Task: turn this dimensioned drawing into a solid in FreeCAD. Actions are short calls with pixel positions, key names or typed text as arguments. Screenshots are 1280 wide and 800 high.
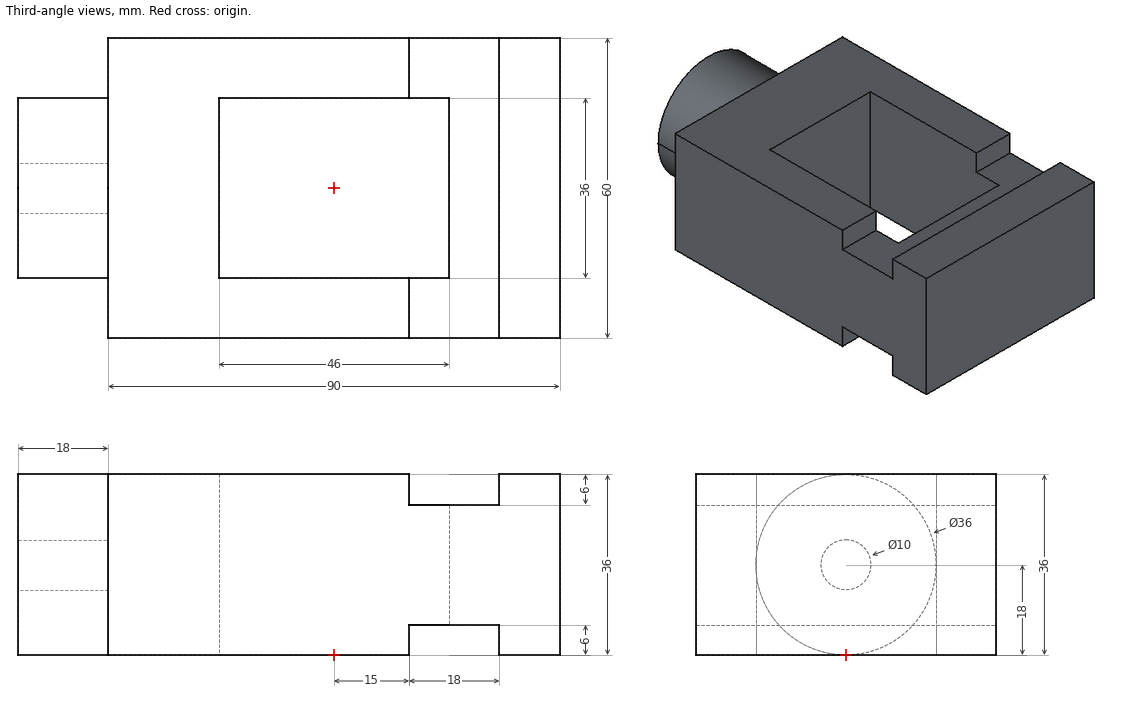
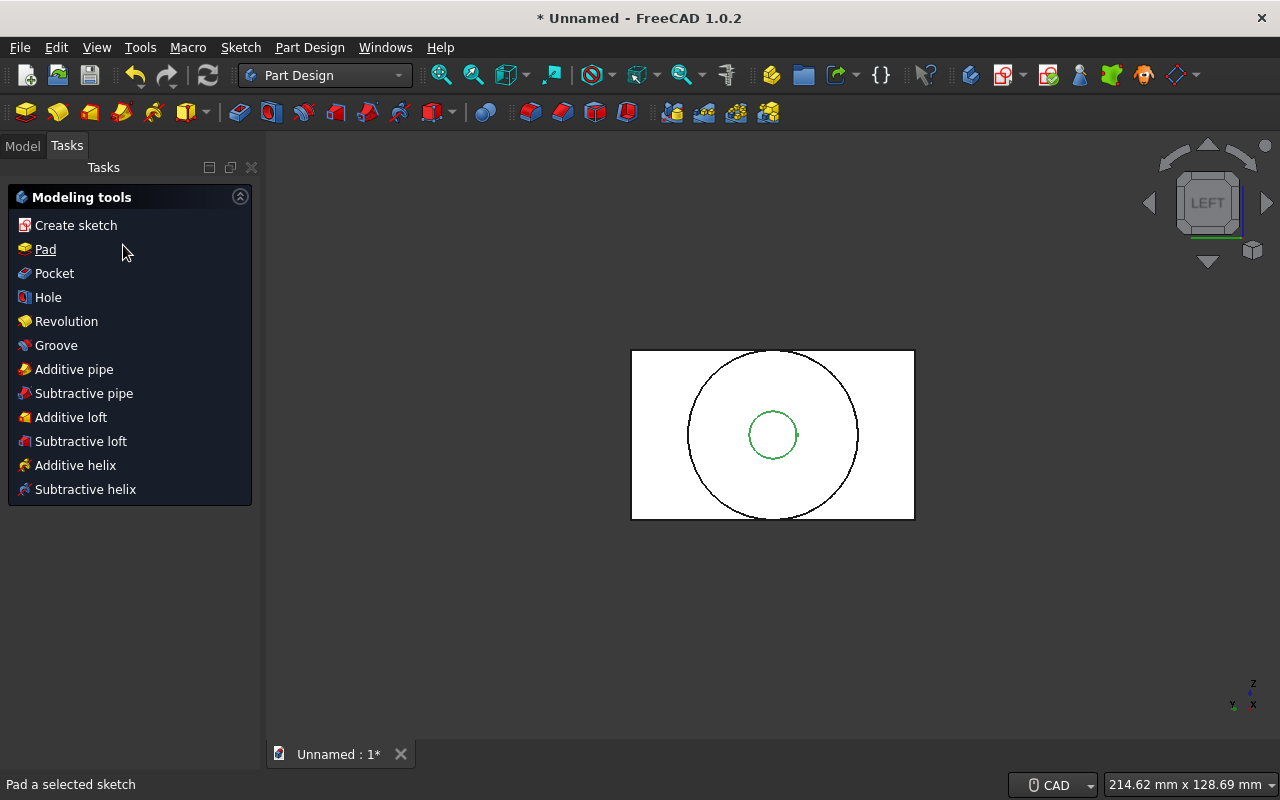
click(240, 112)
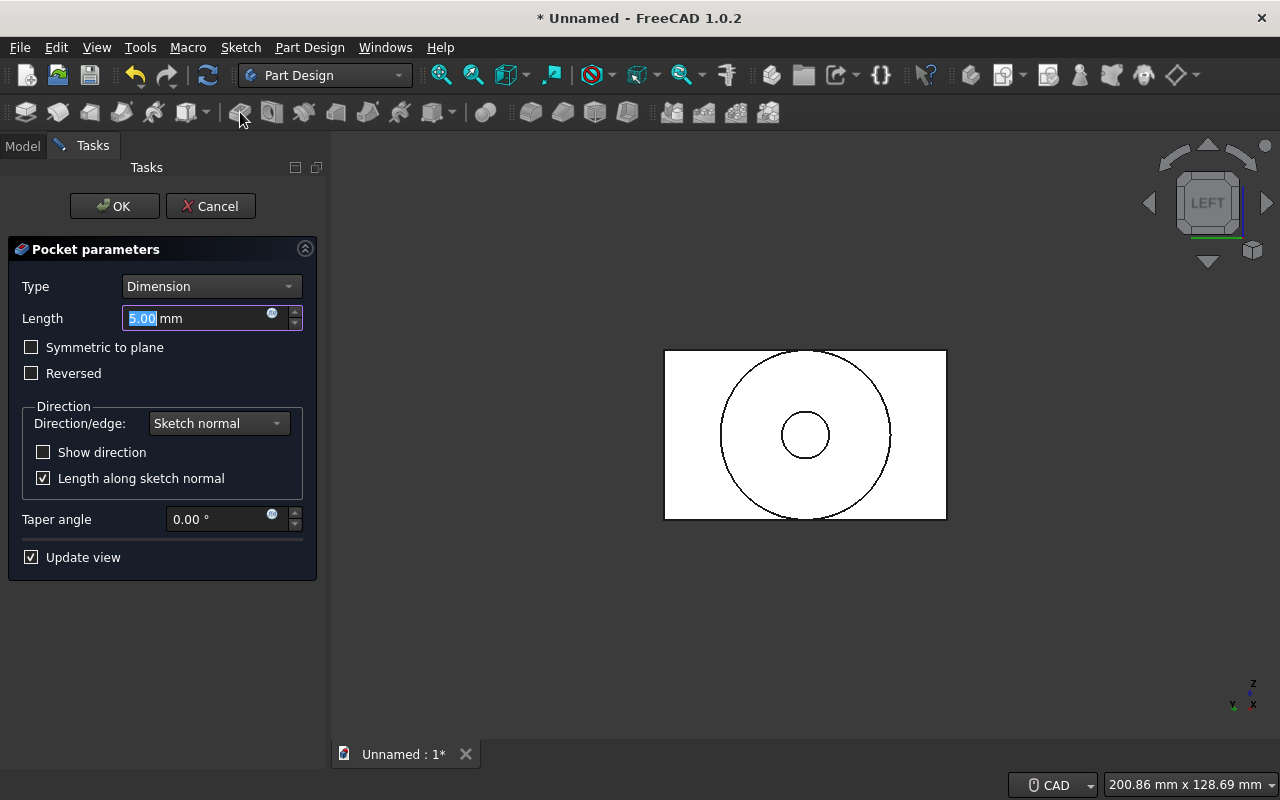
text(18)
key(Tab)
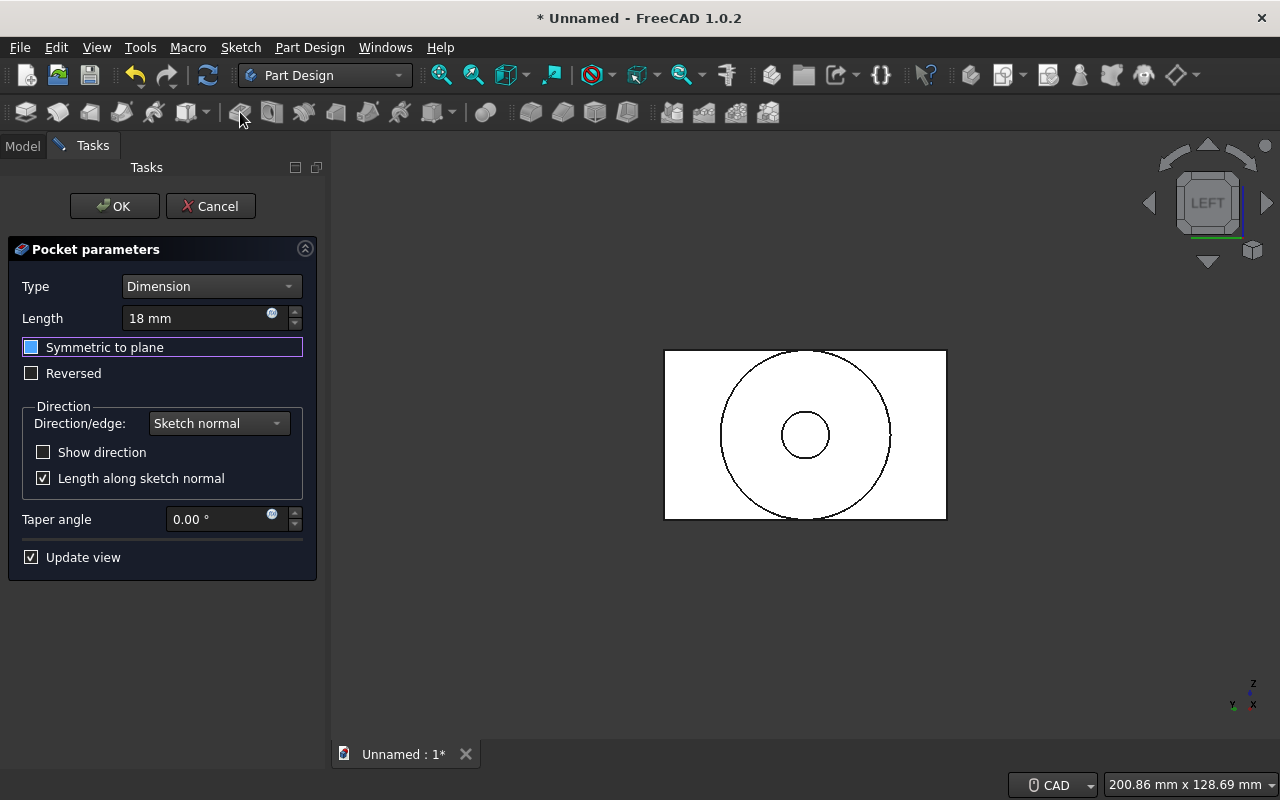
click(115, 206)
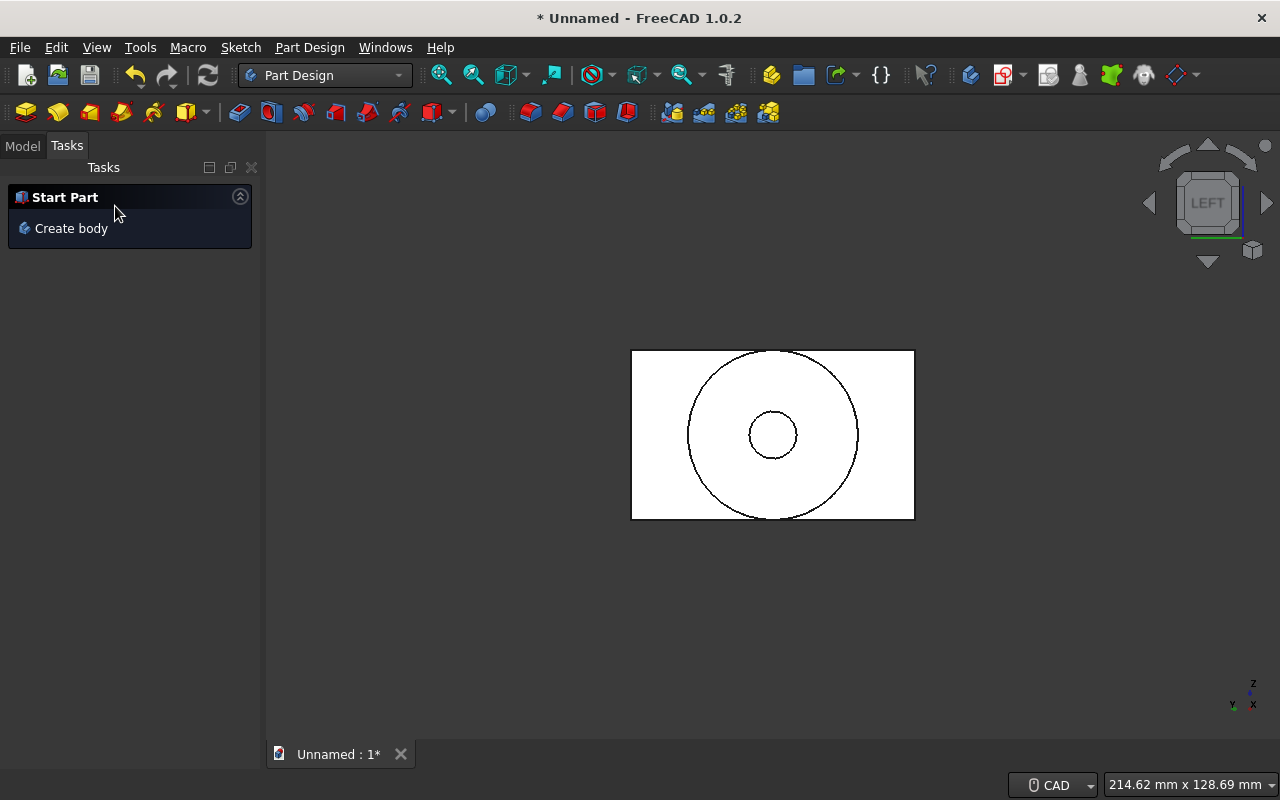
click(442, 76)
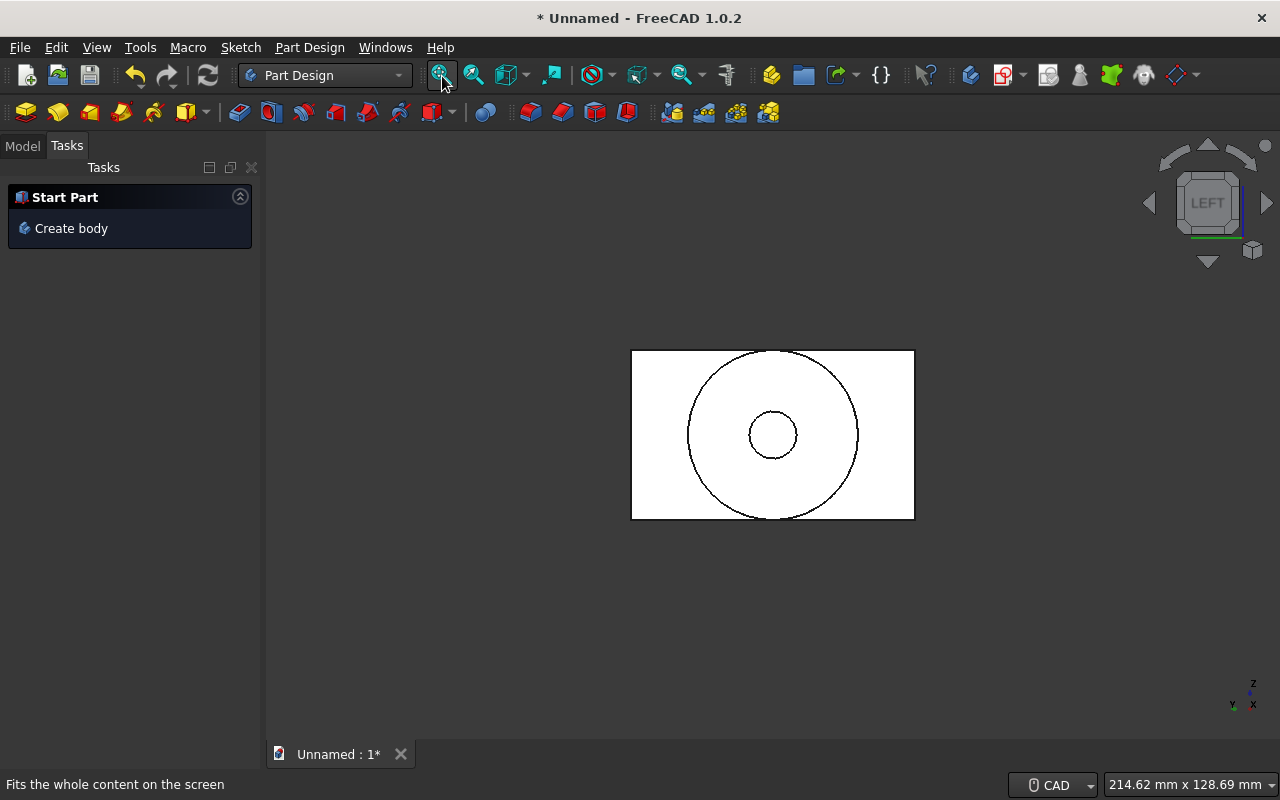
key(0)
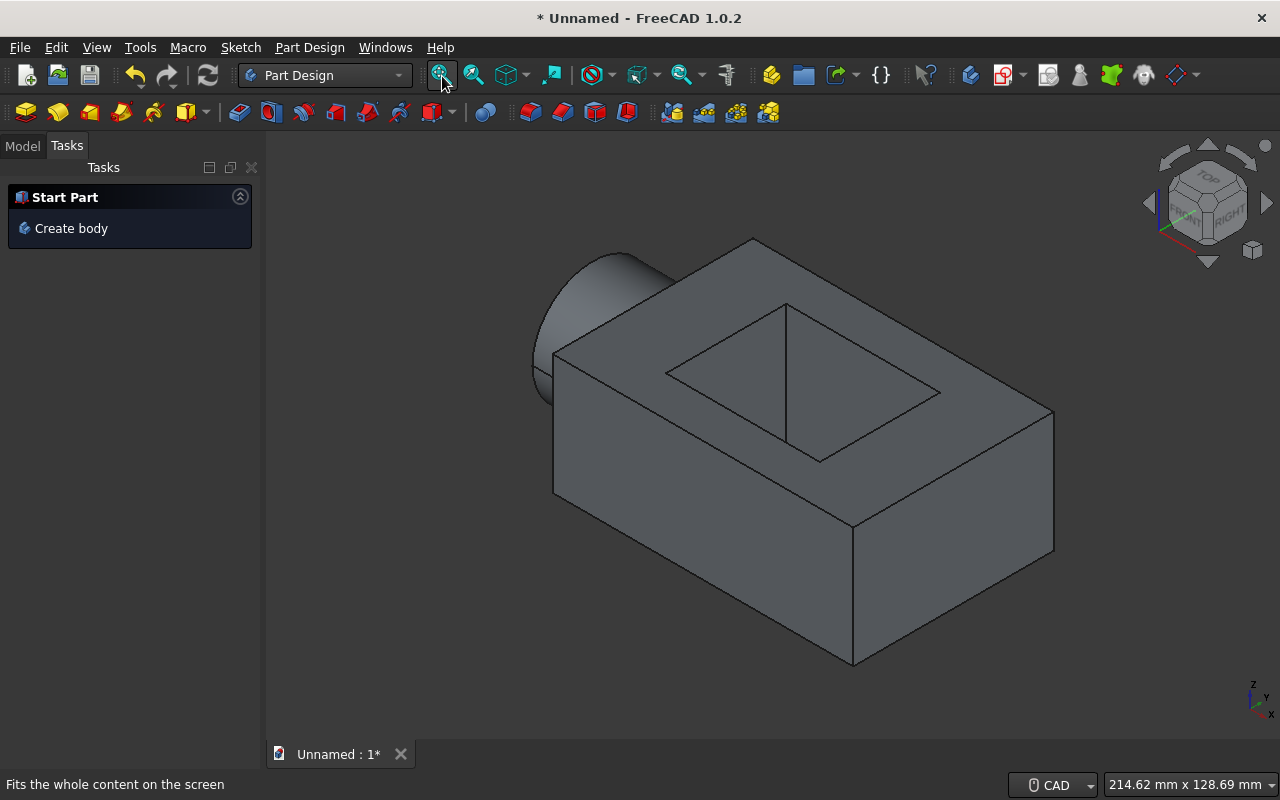
click(789, 559)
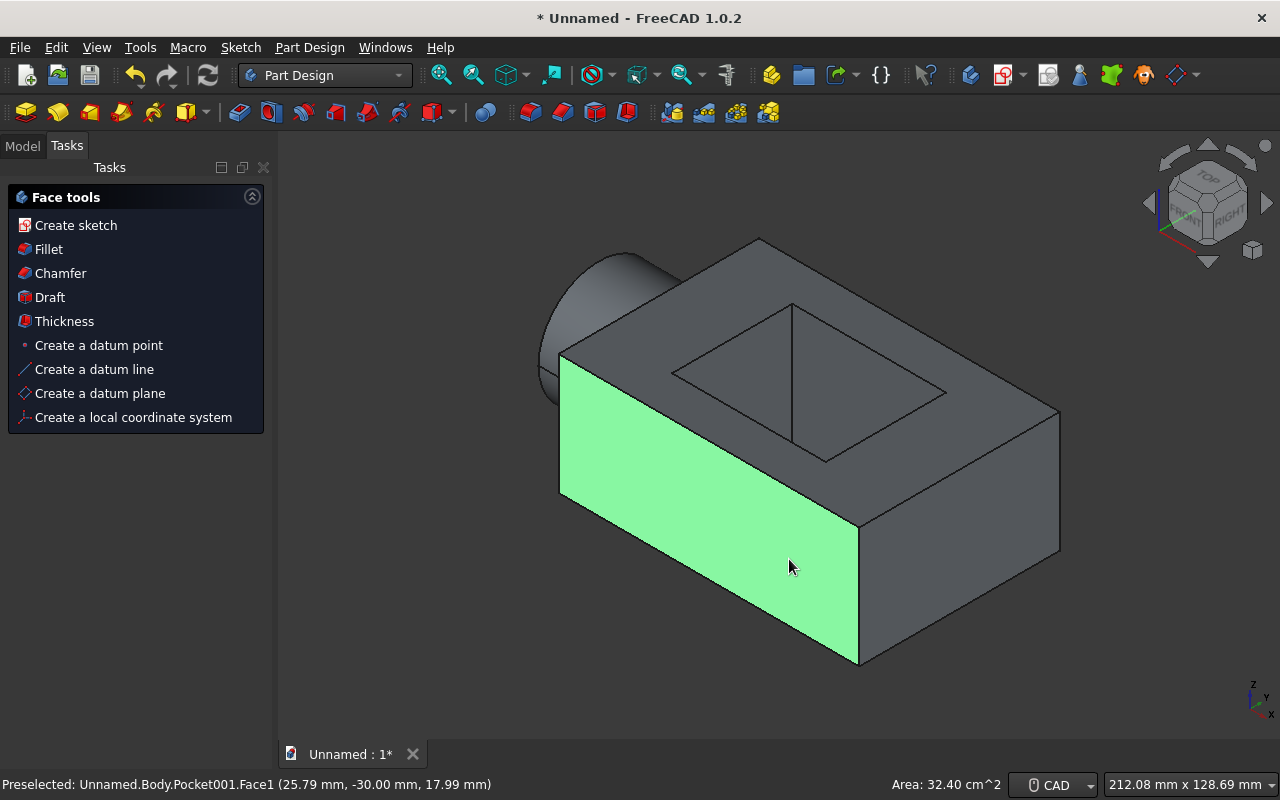
click(1004, 76)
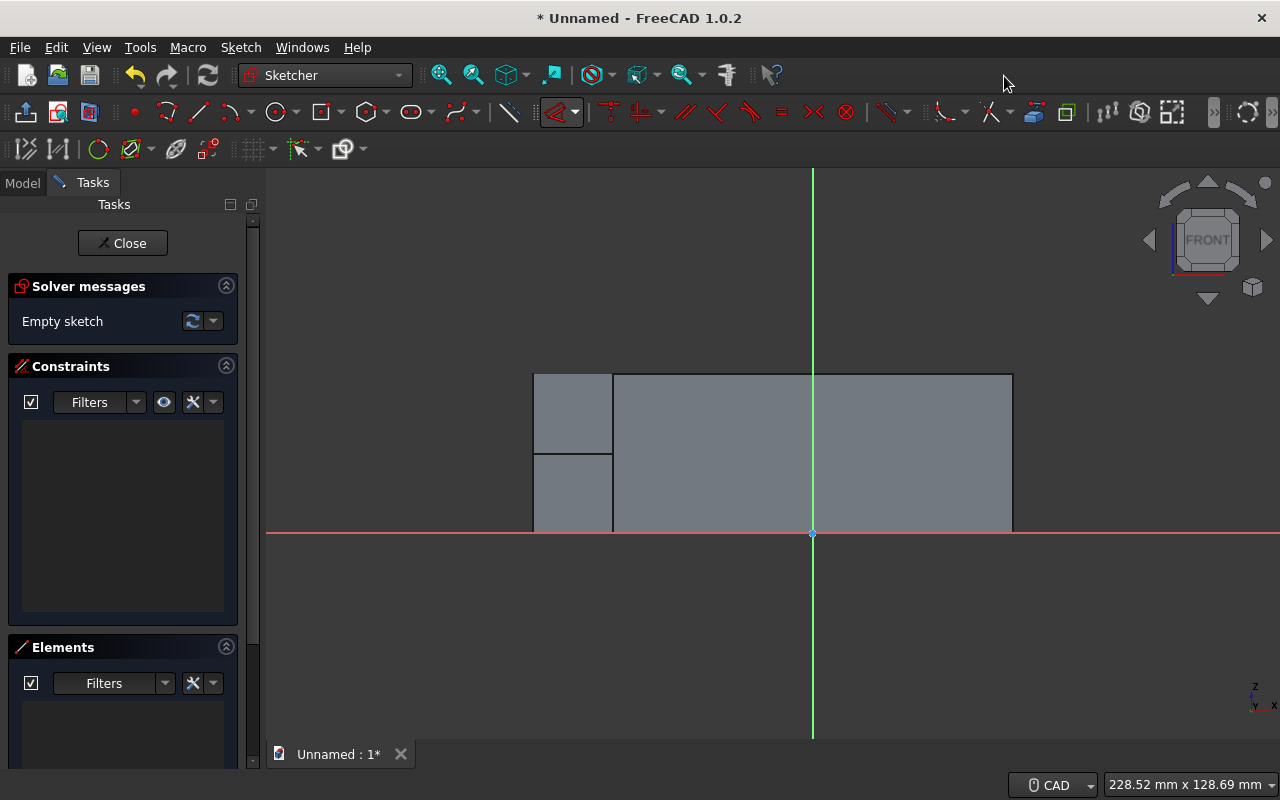
scroll(946, 542, up, 7)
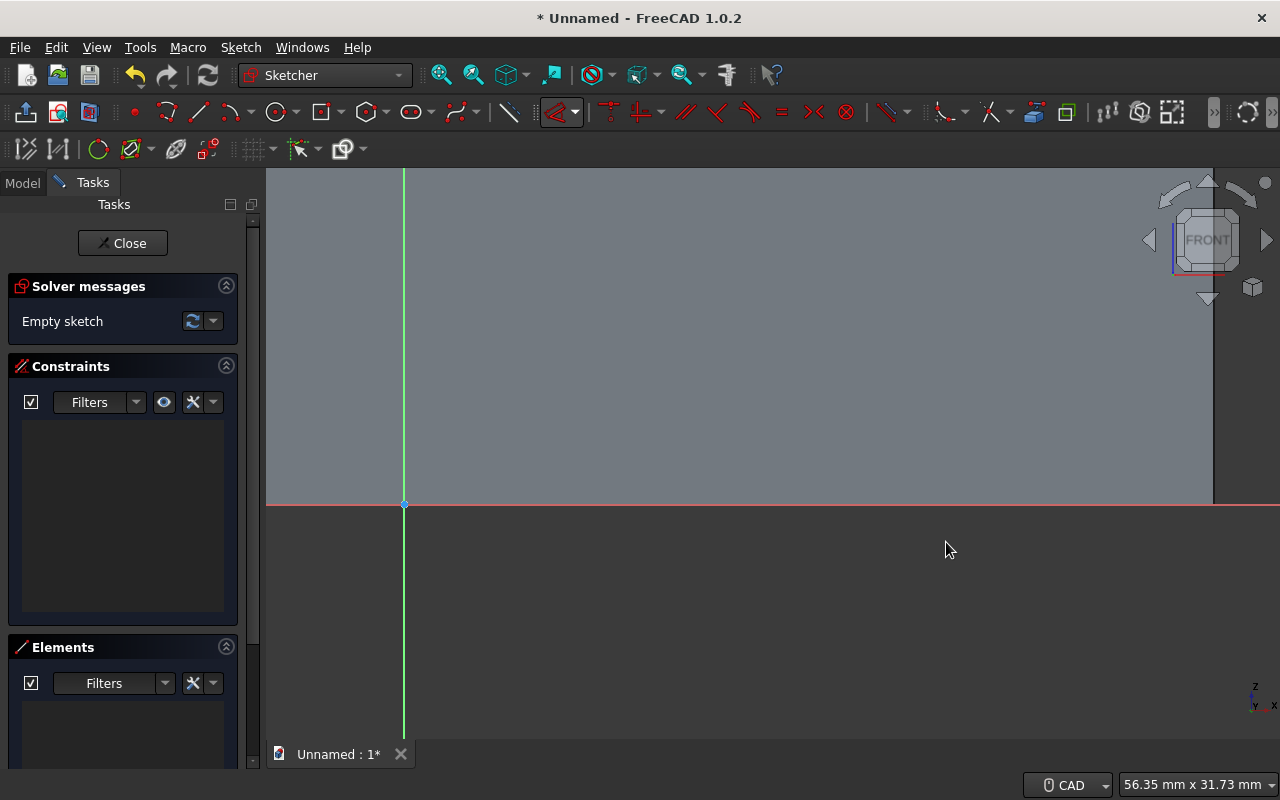
key(g)
key(r)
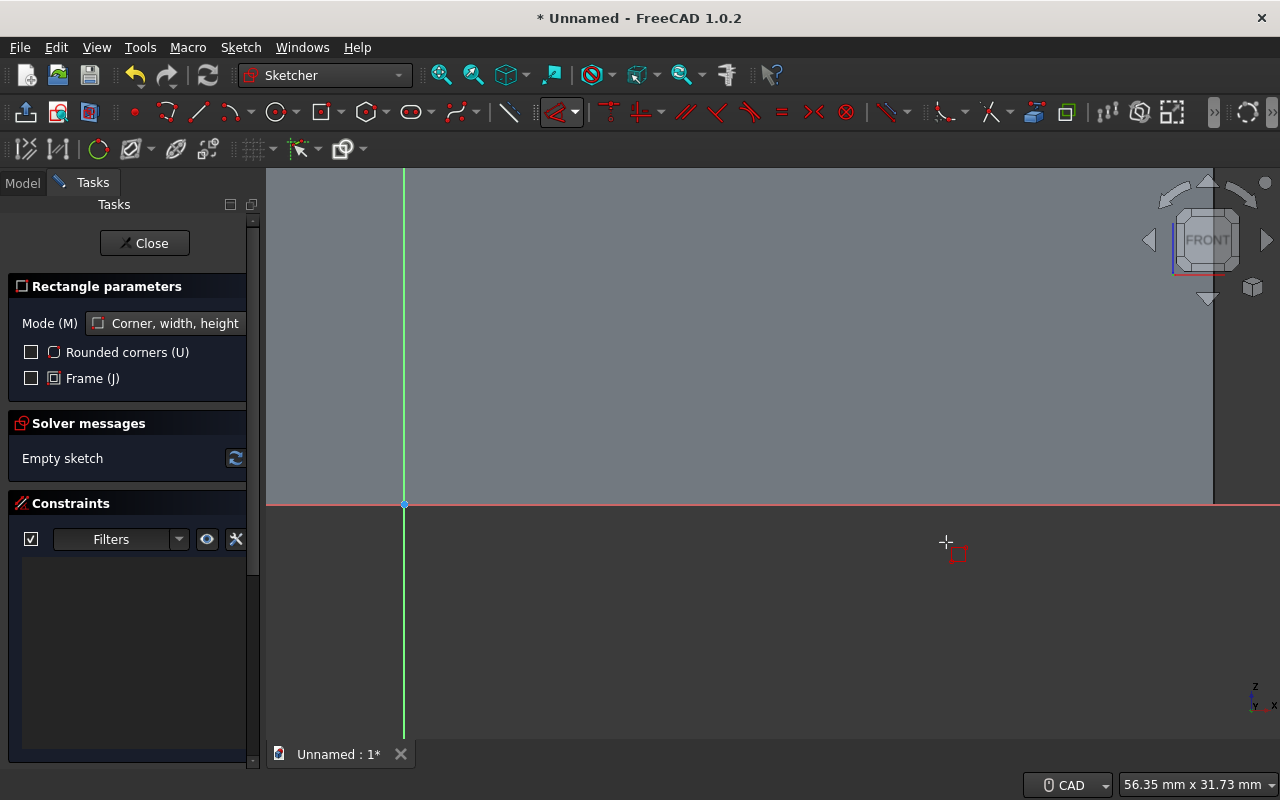
click(674, 397)
click(998, 505)
key(Escape)